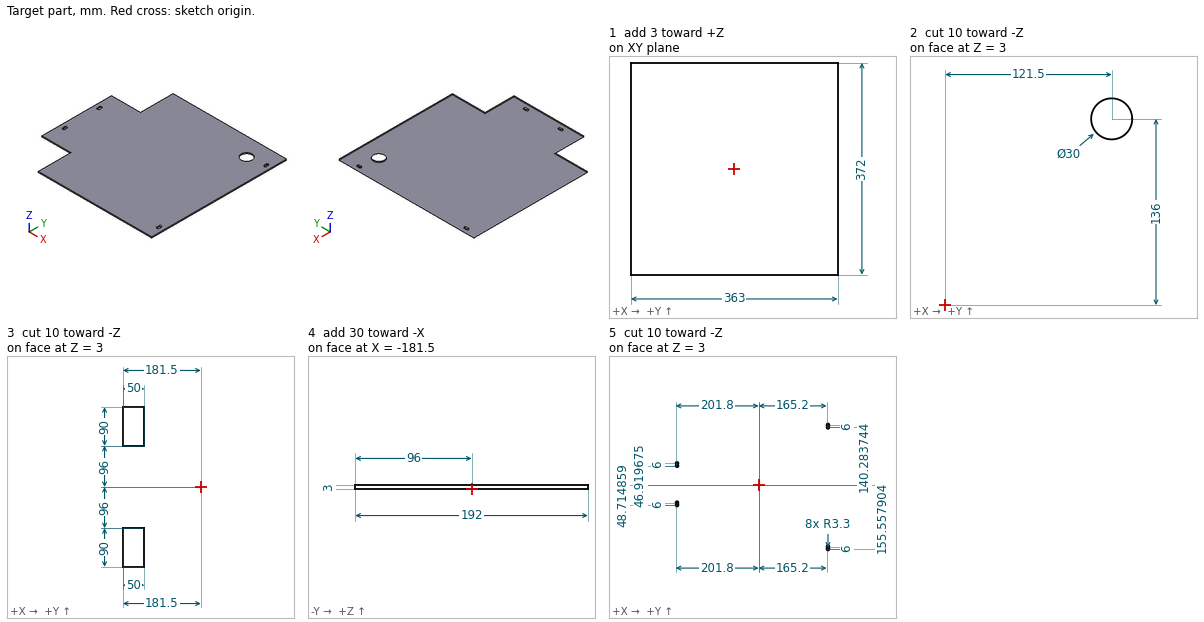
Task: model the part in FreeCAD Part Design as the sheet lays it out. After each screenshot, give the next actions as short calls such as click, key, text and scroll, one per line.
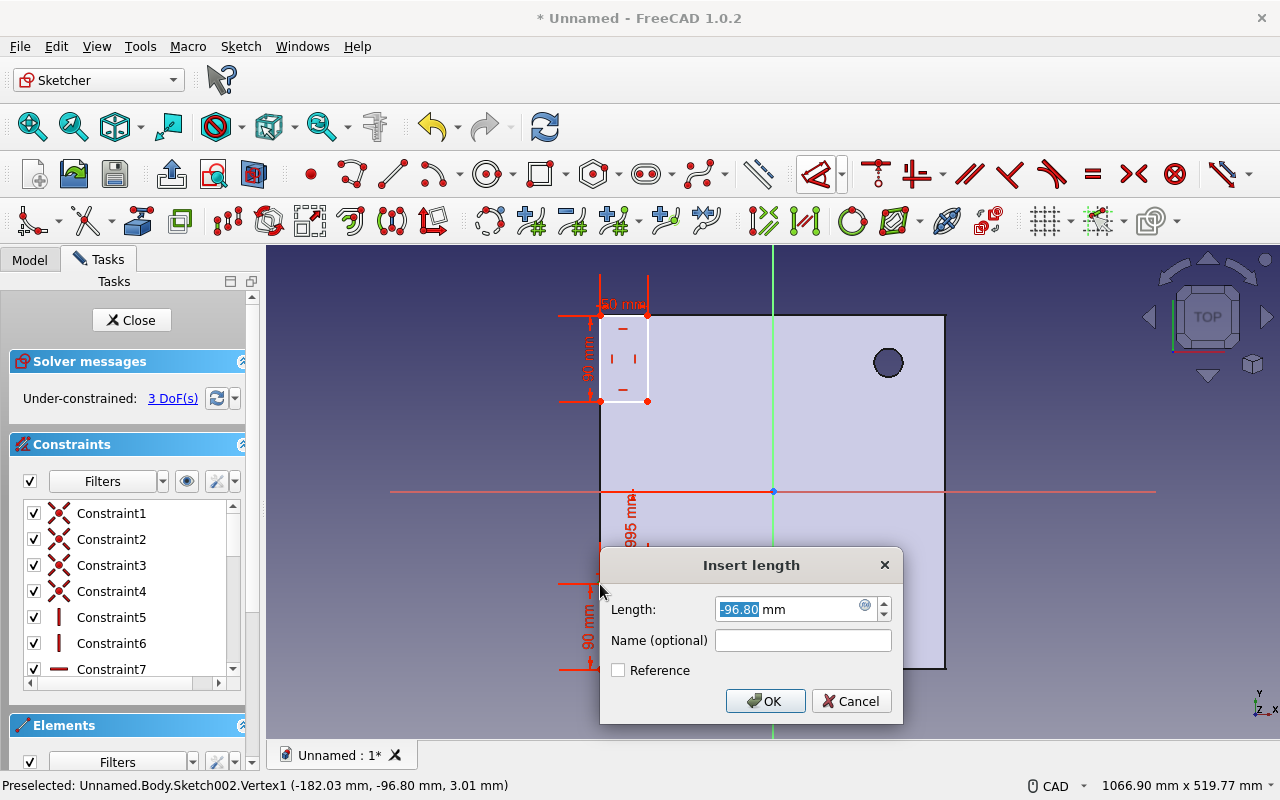
text(-96)
key(Return)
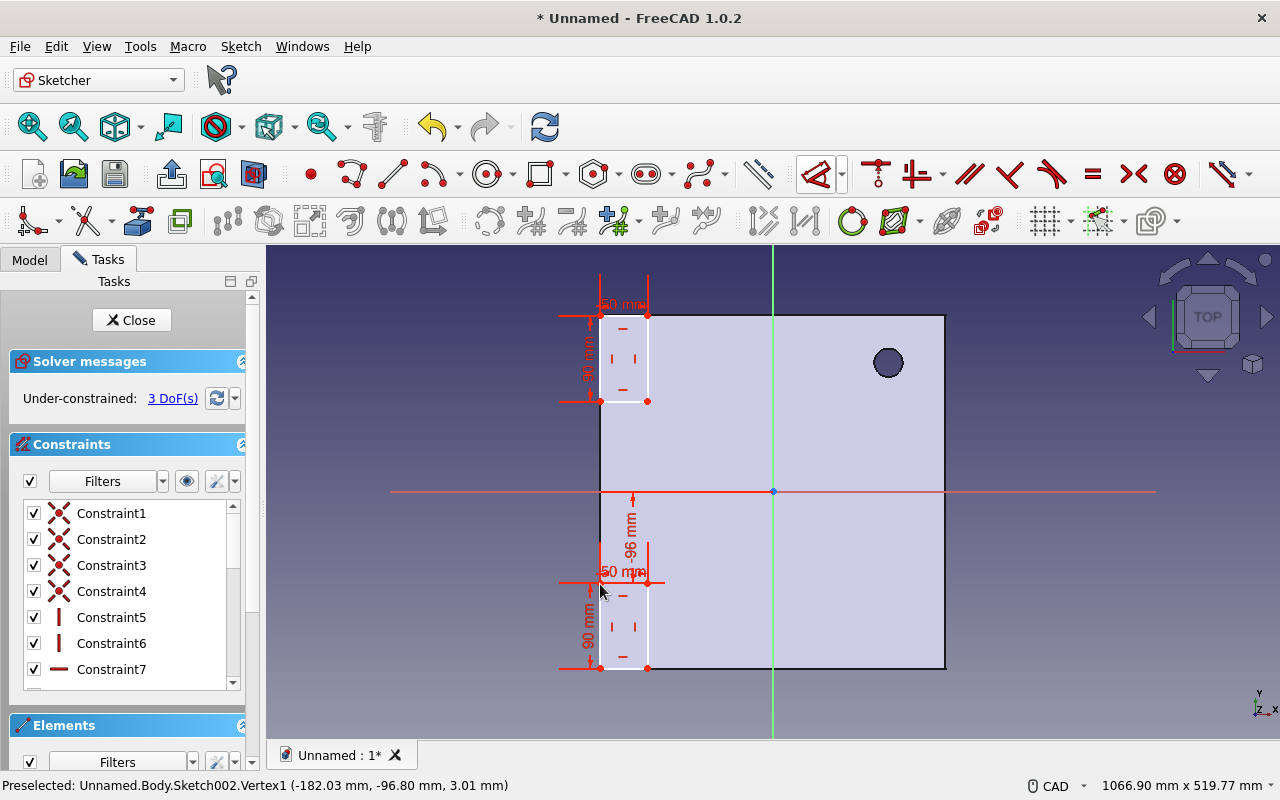
click(600, 402)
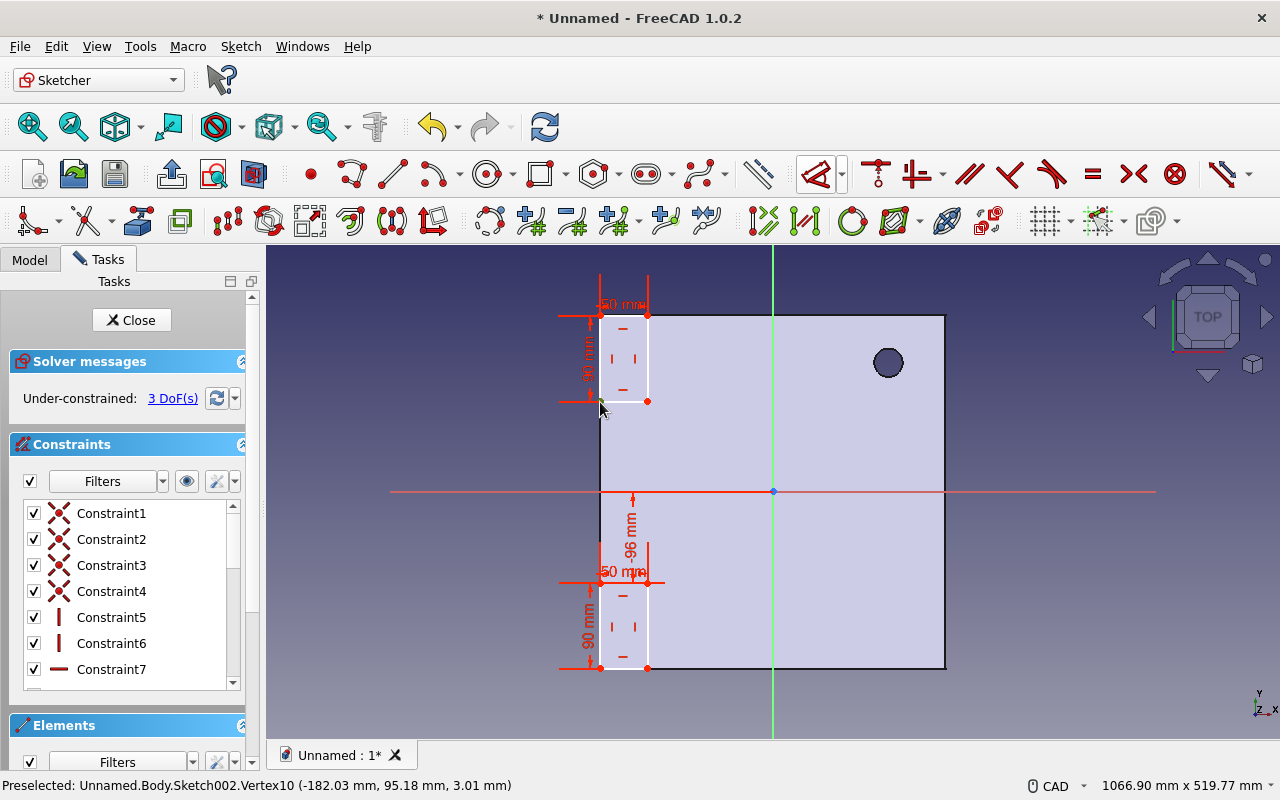
click(842, 174)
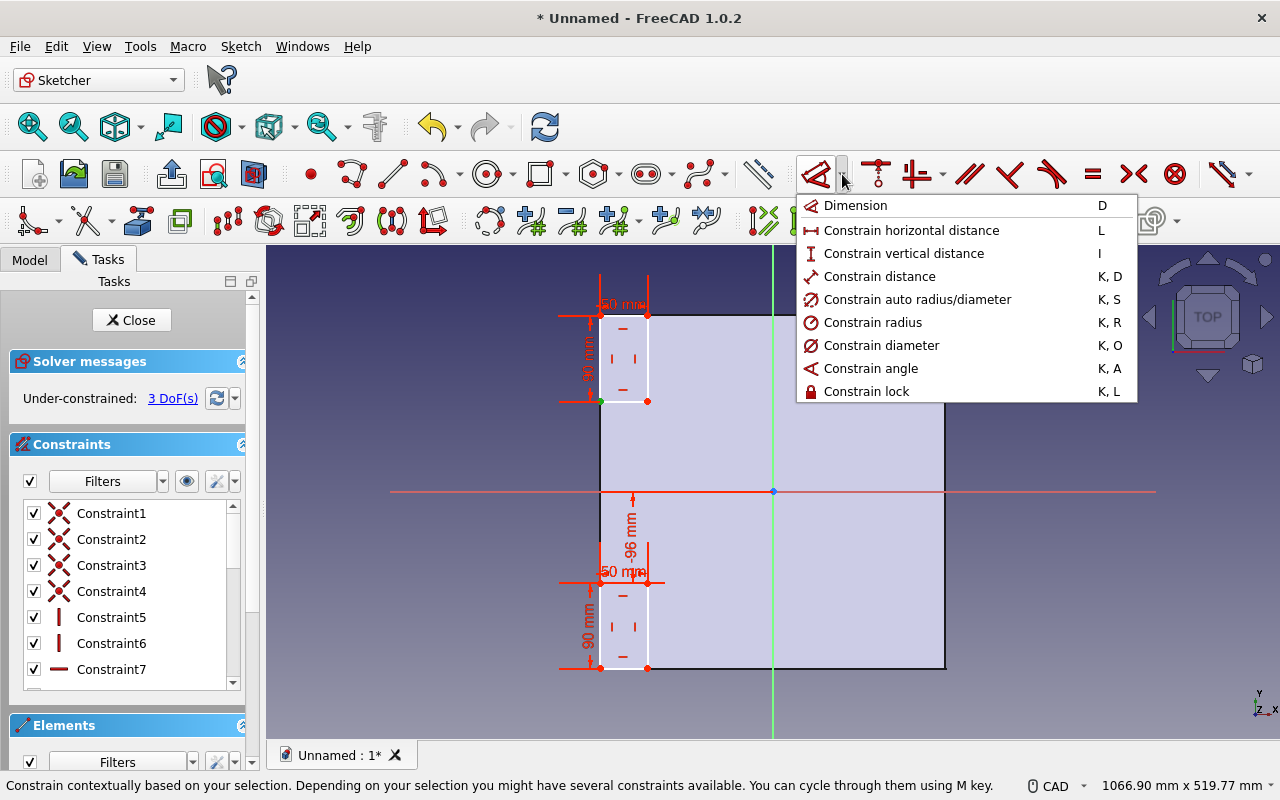
click(967, 254)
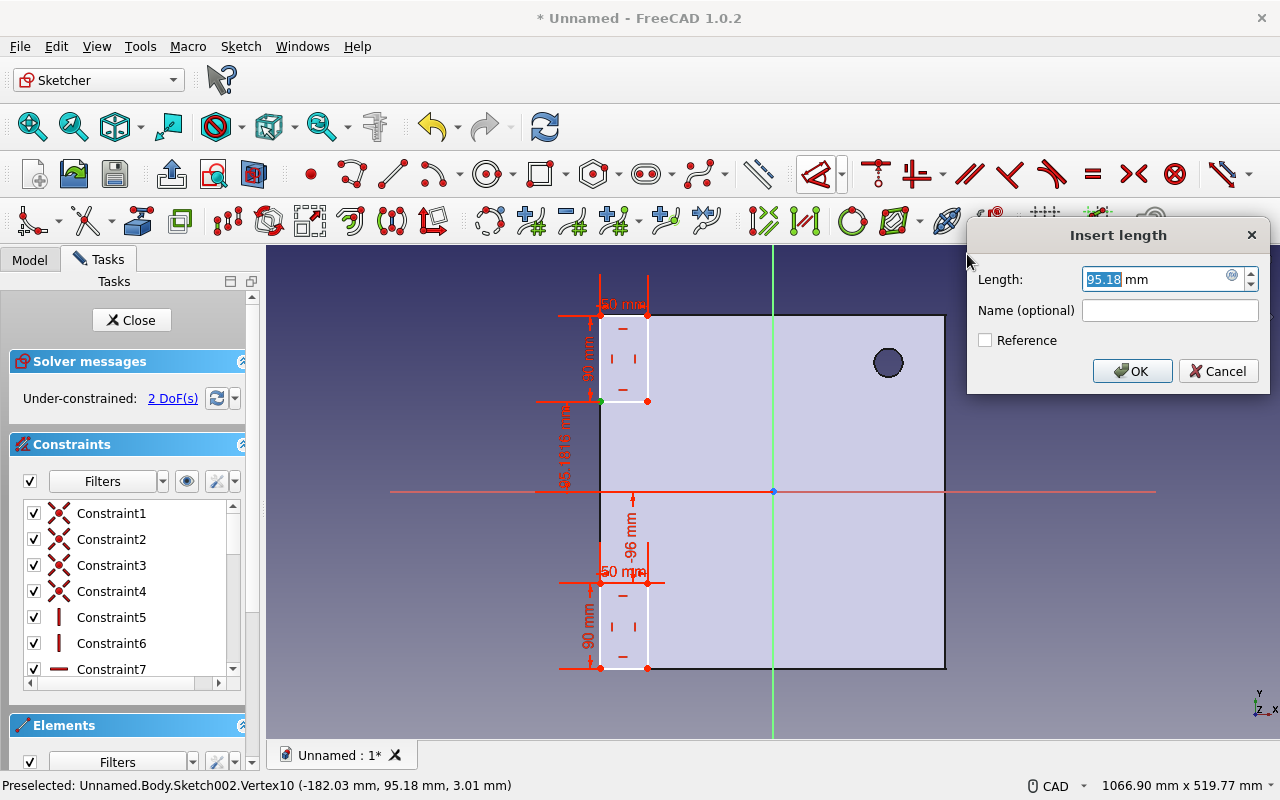
text(96)
key(Return)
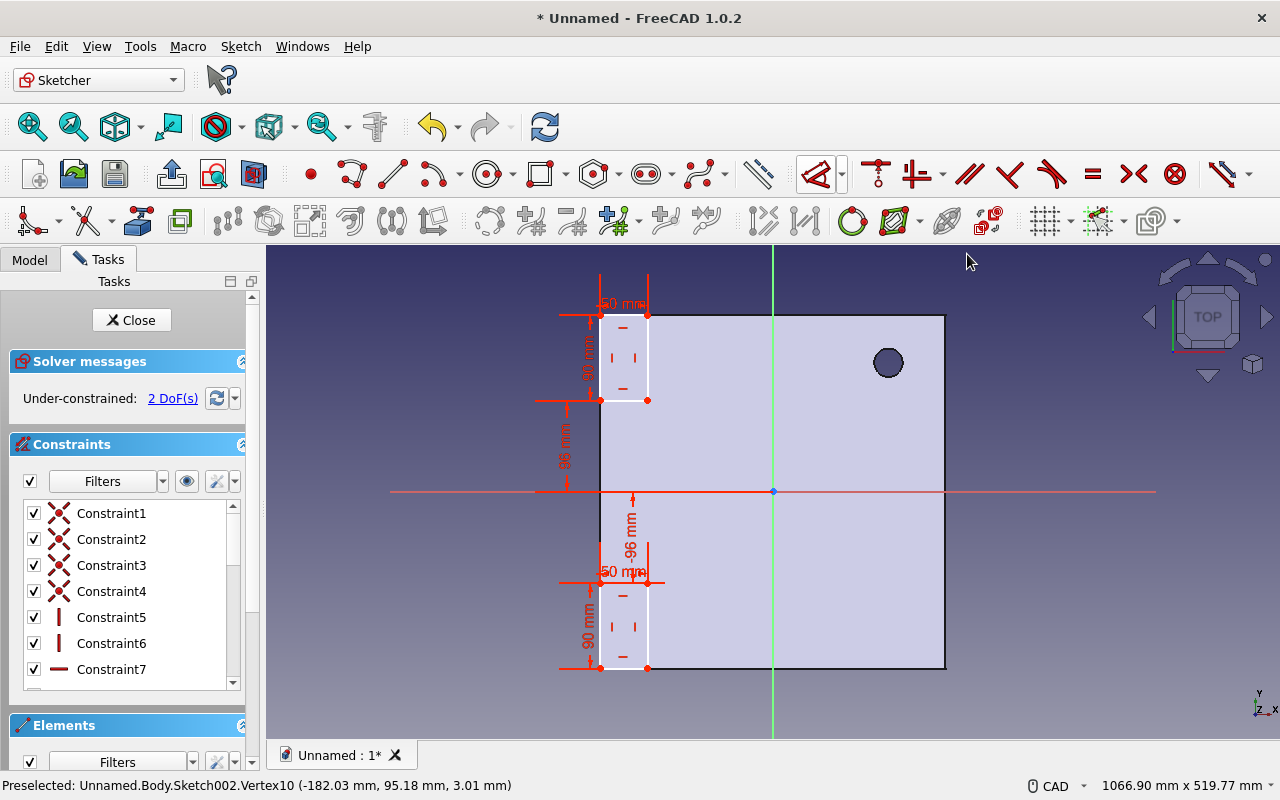
click(600, 583)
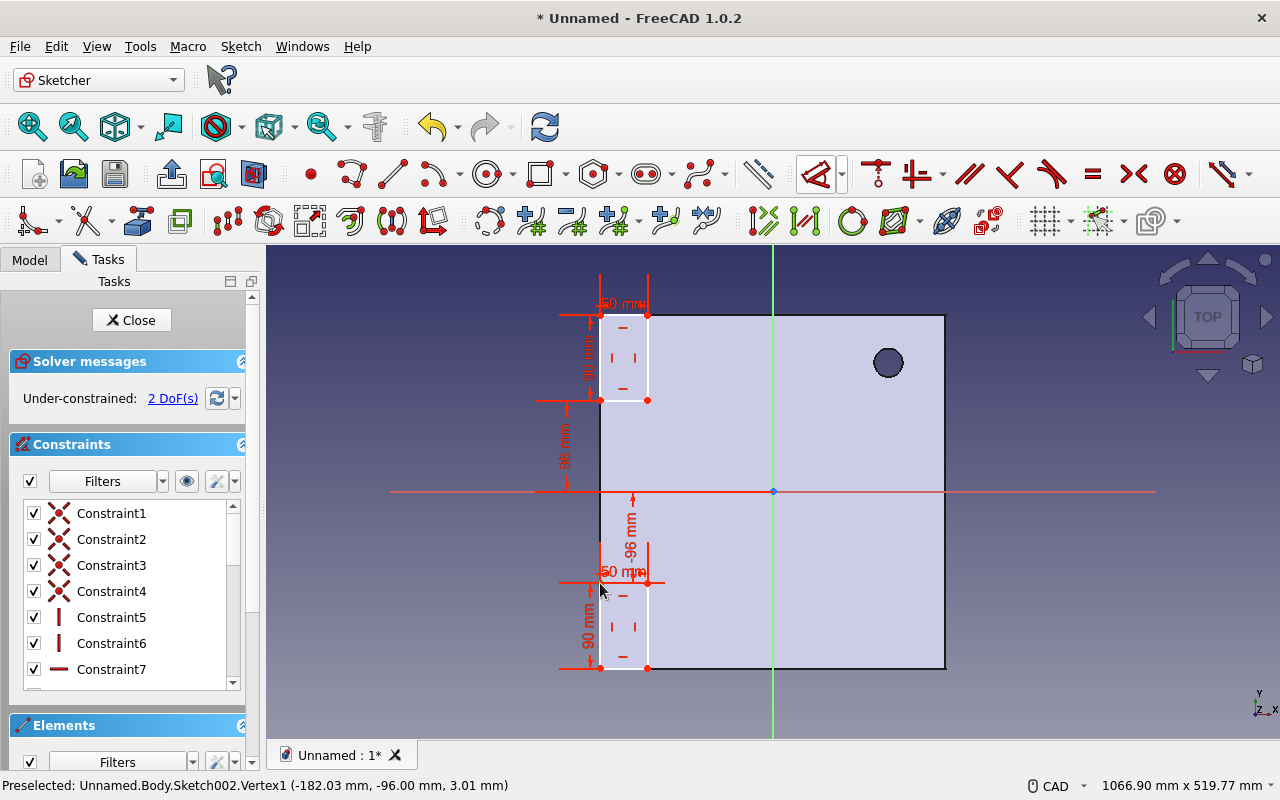
key(l)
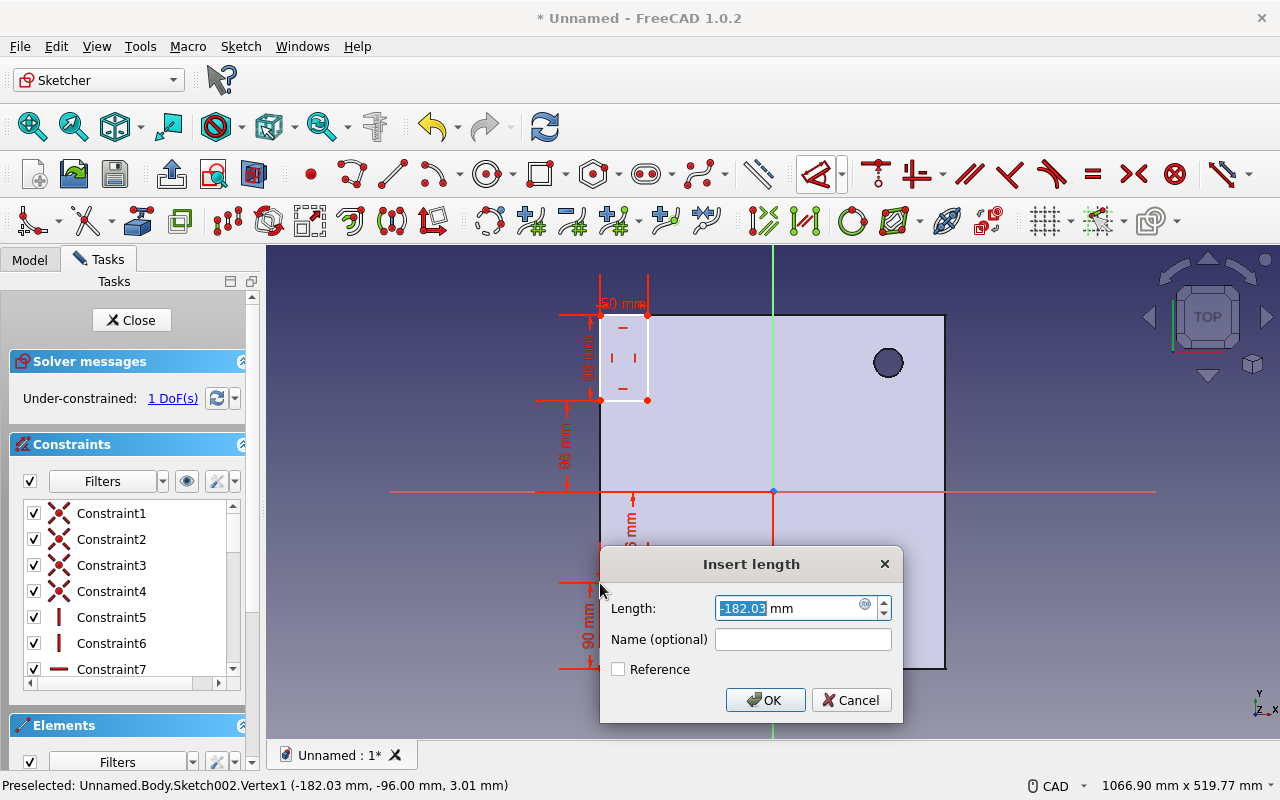
text(-181.5)
key(Return)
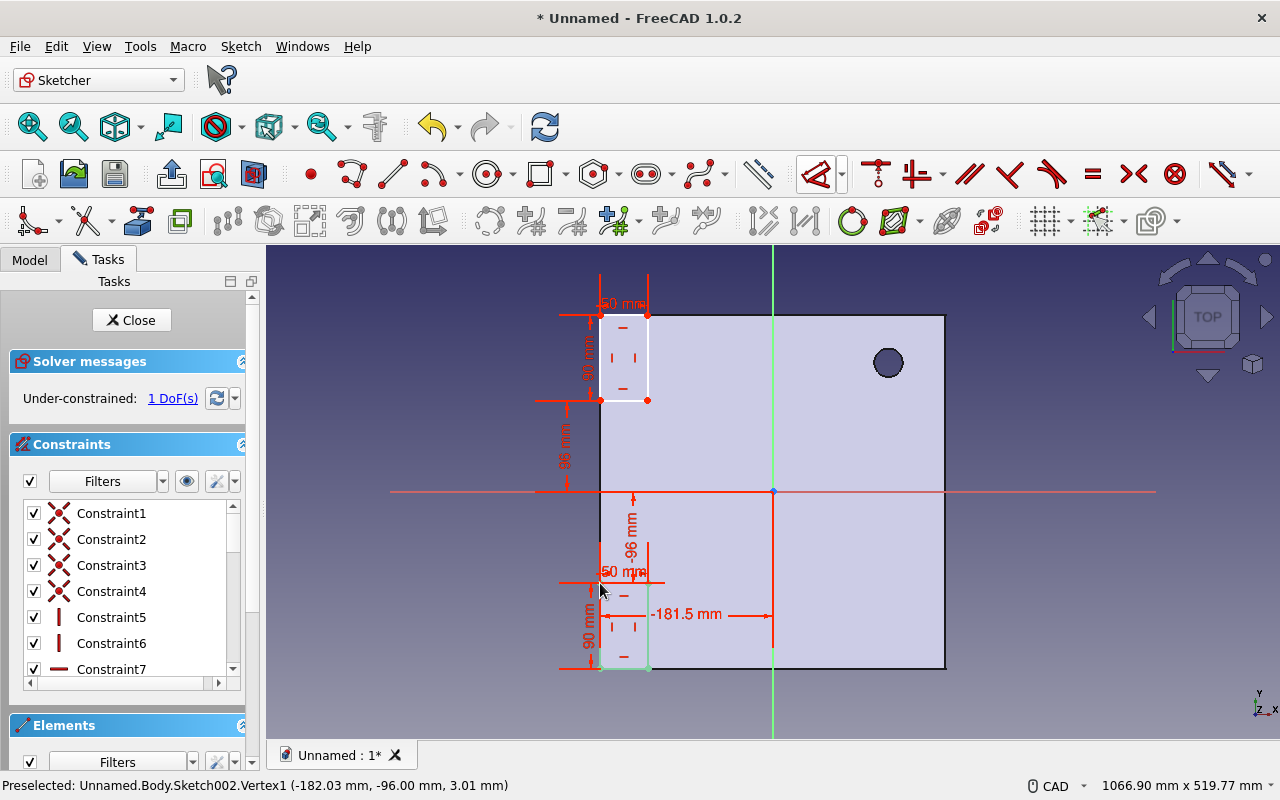
click(600, 315)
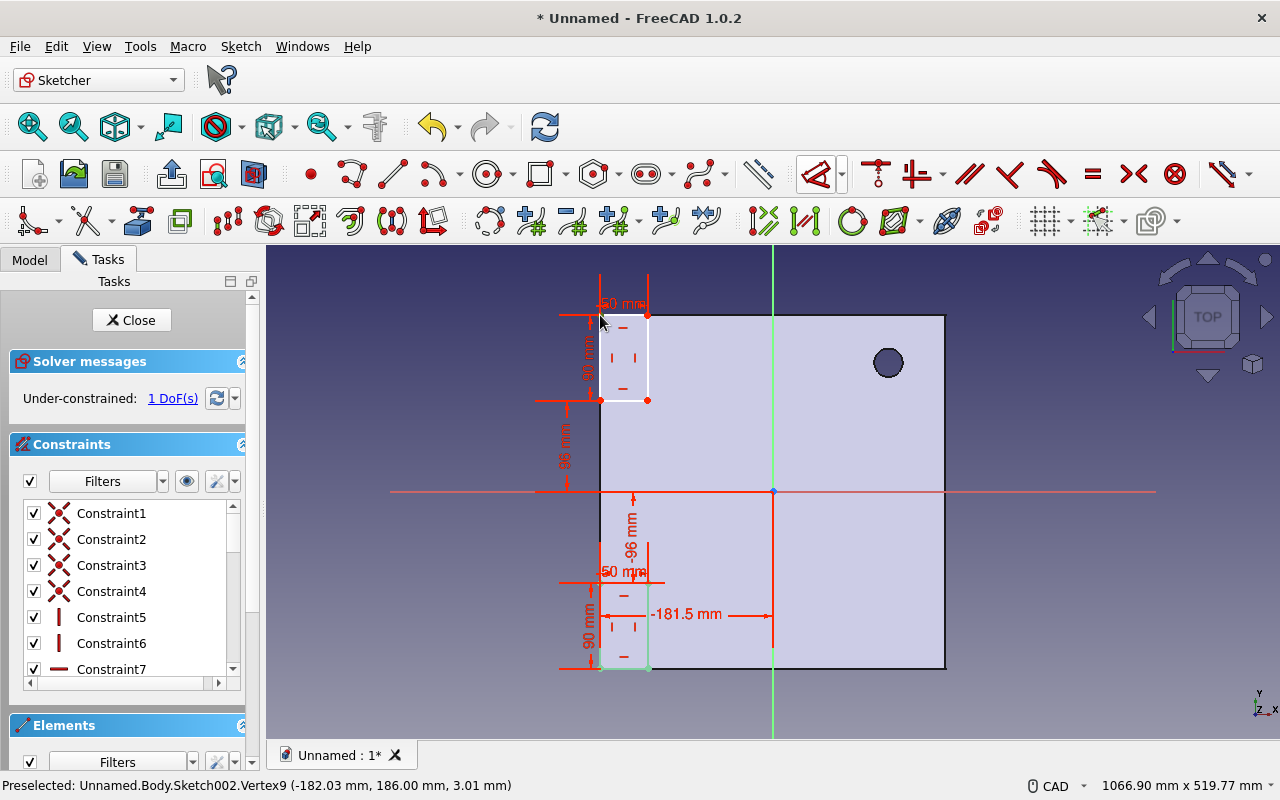
key(l)